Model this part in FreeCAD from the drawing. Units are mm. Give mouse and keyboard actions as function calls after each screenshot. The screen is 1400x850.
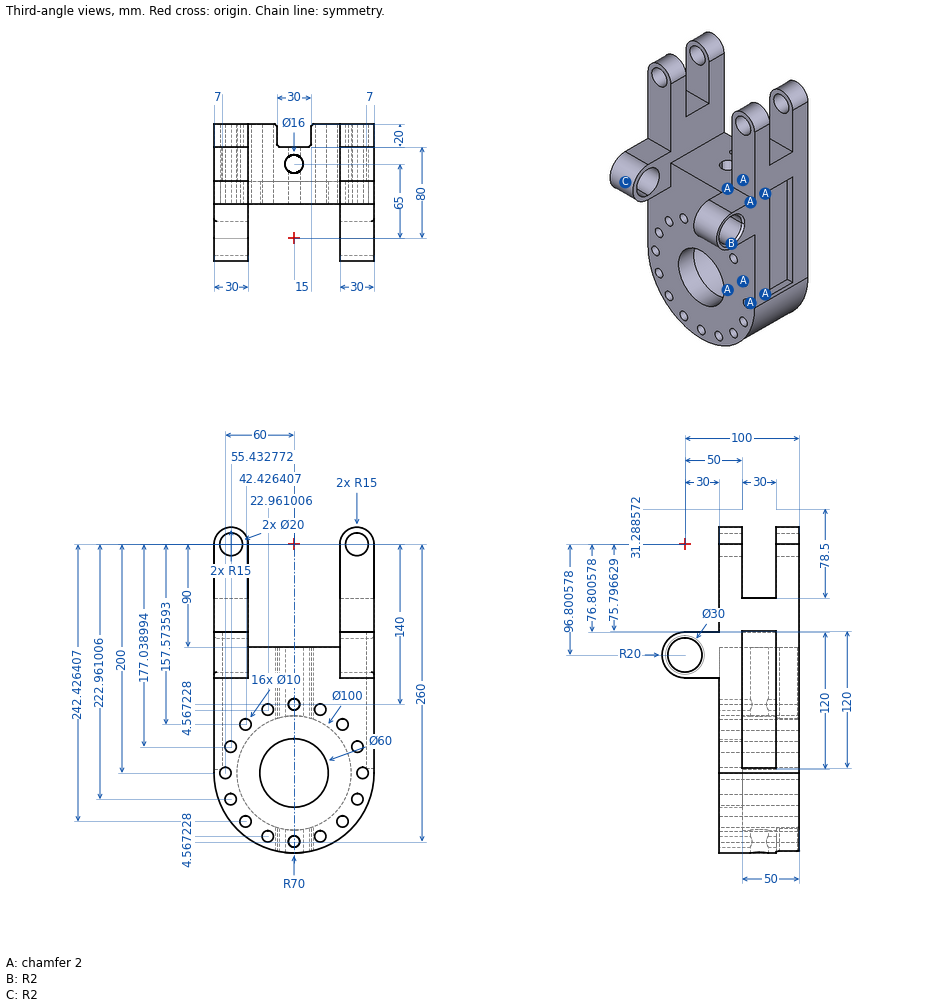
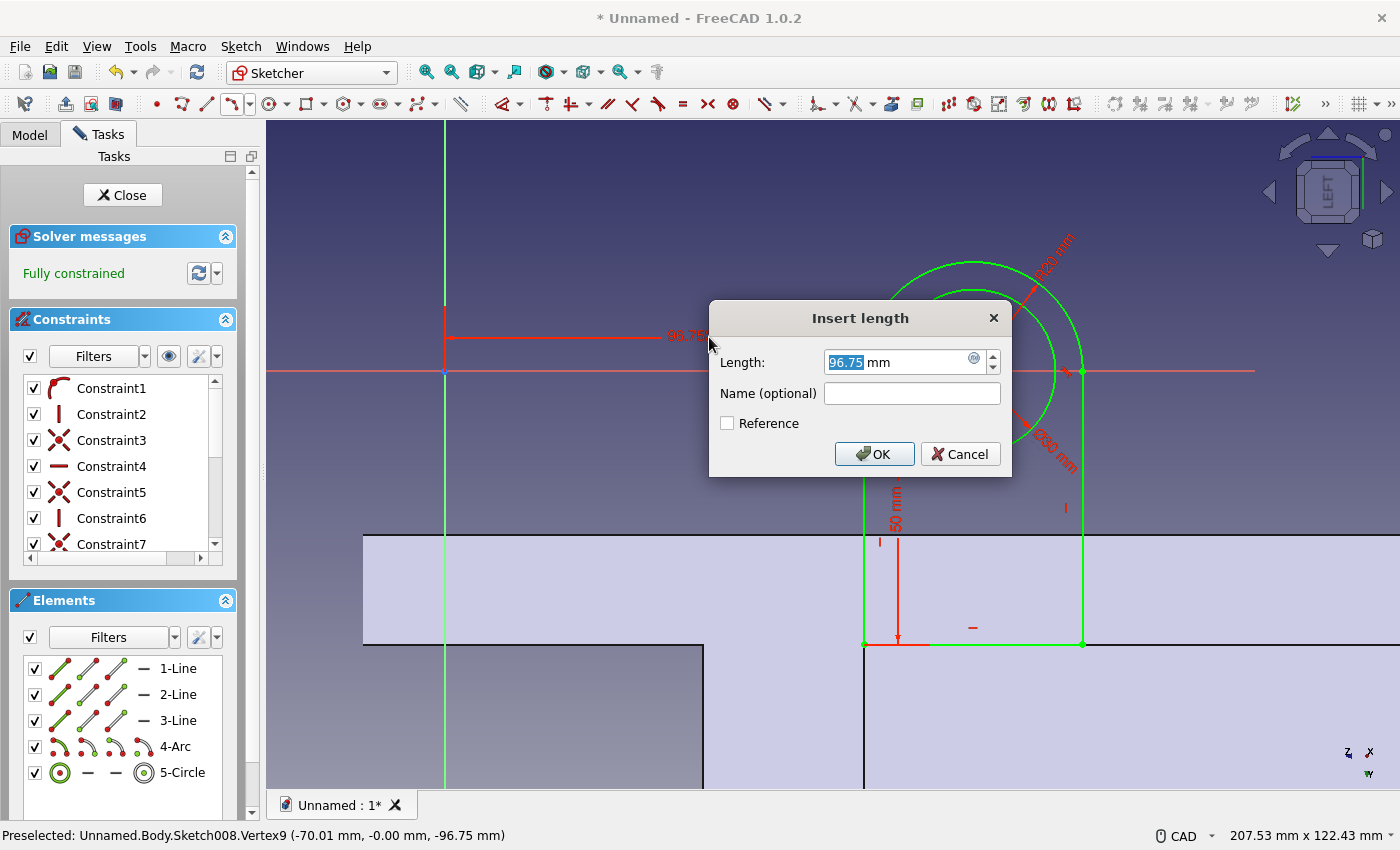
text(96.800578)
key(Return)
key(Escape)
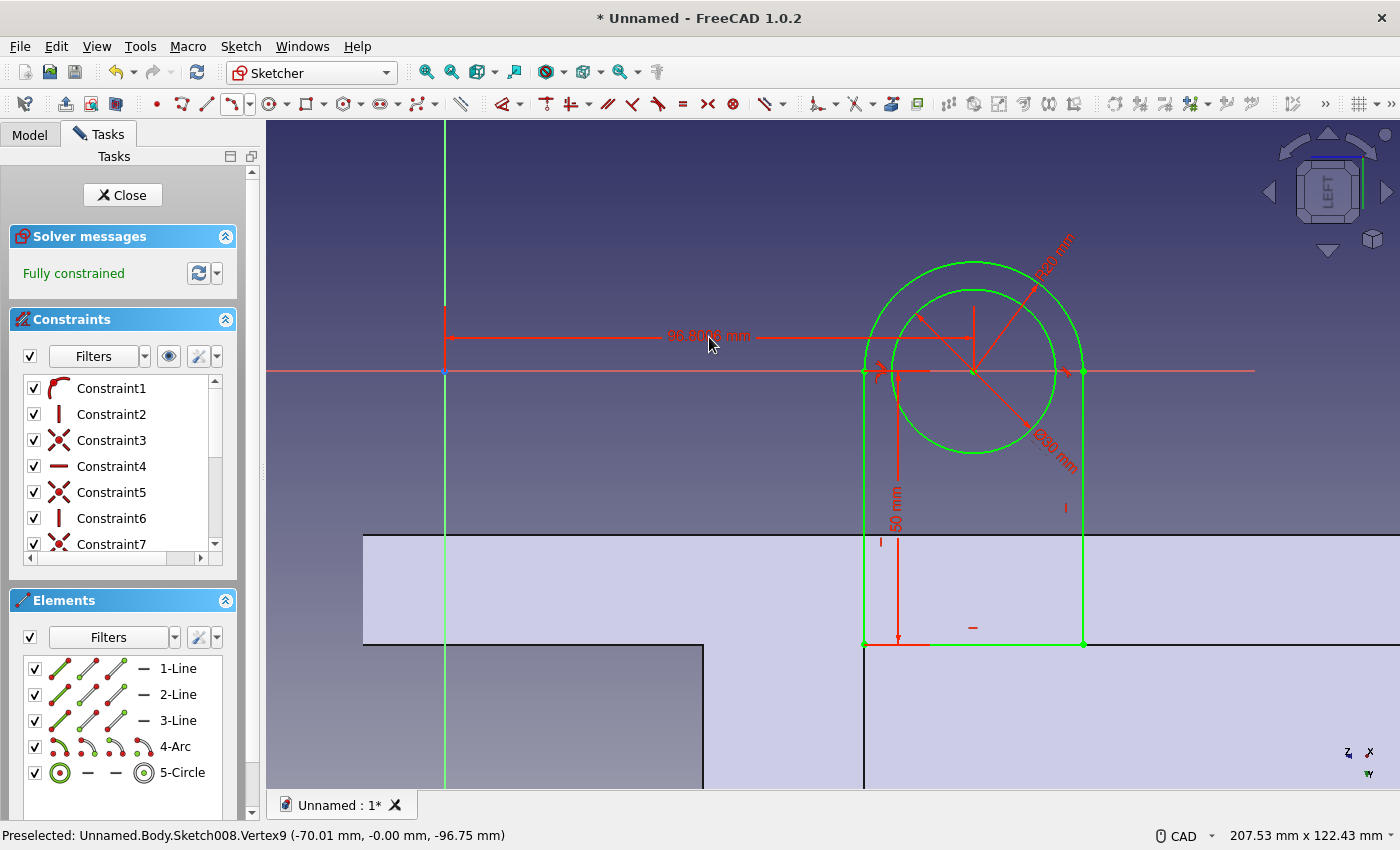
click(123, 195)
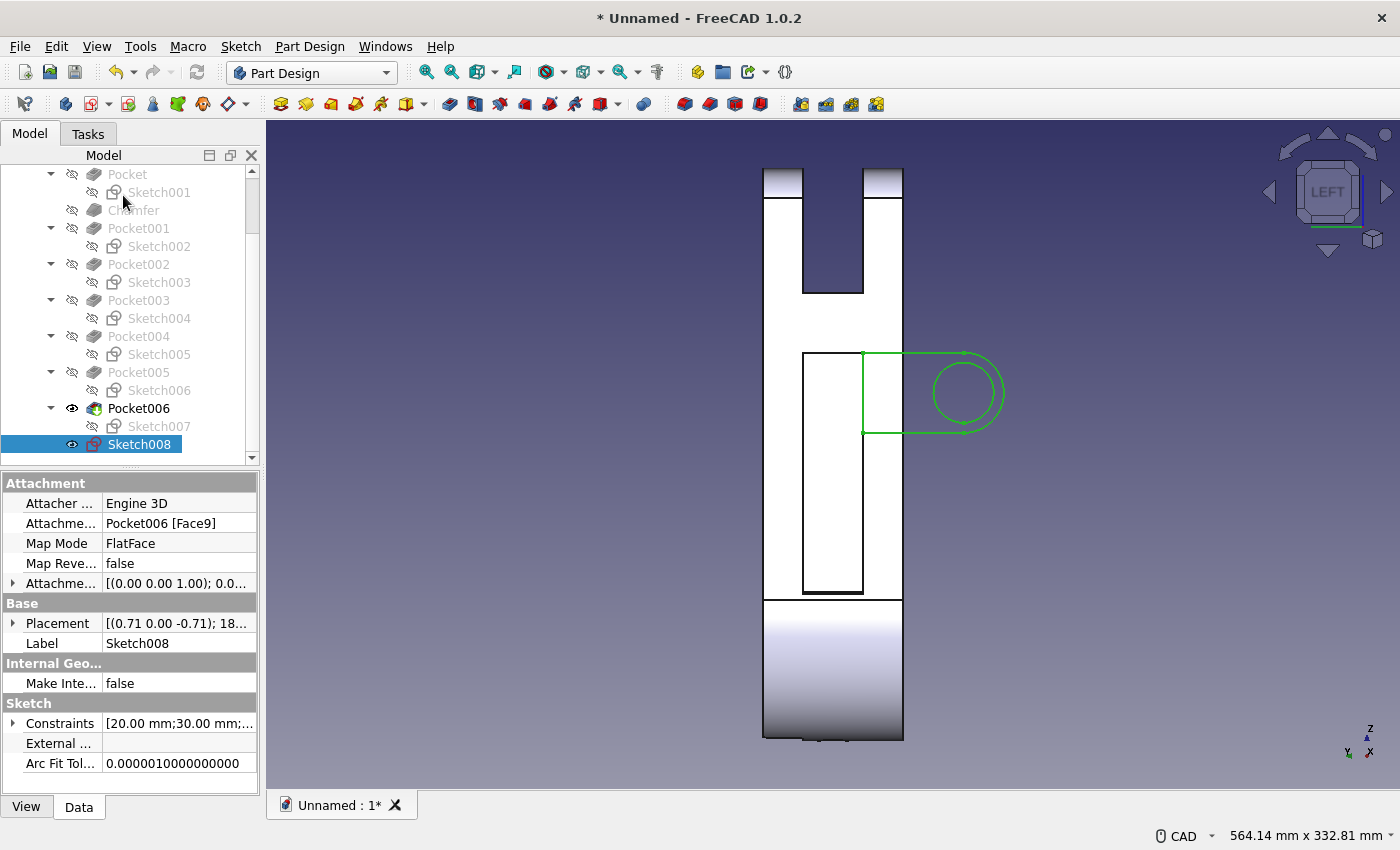
click(281, 104)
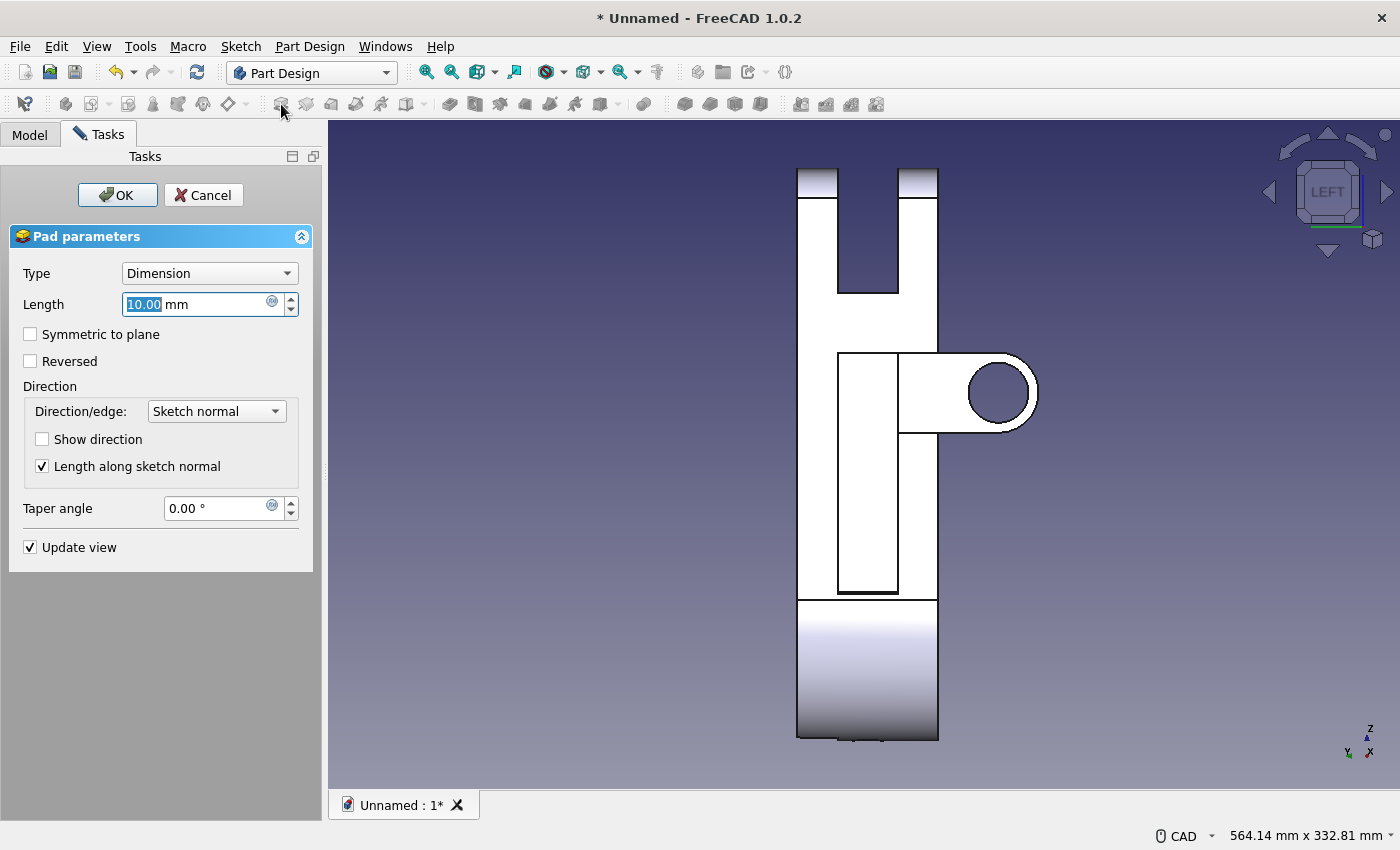
text(30)
key(Tab)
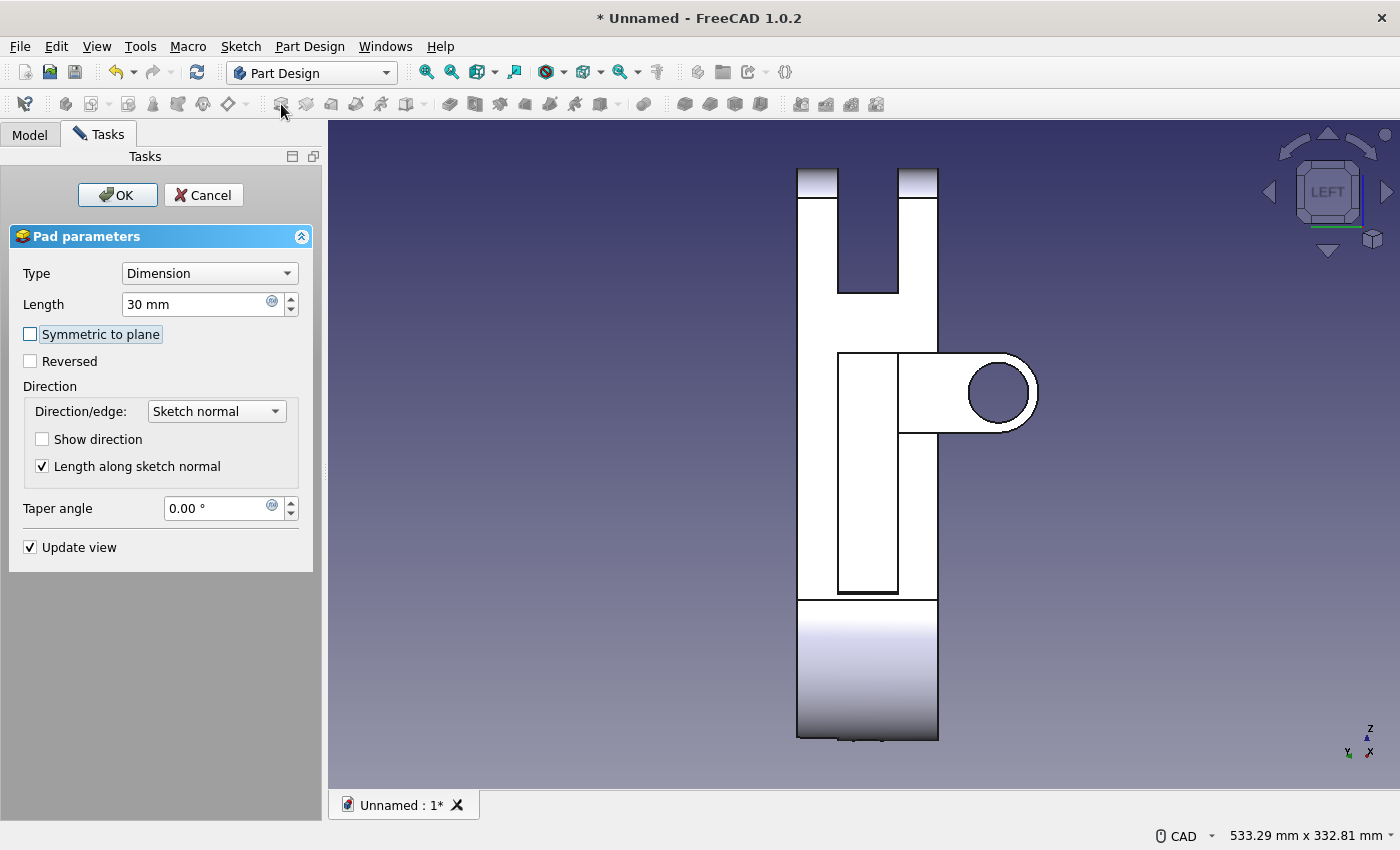
click(31, 361)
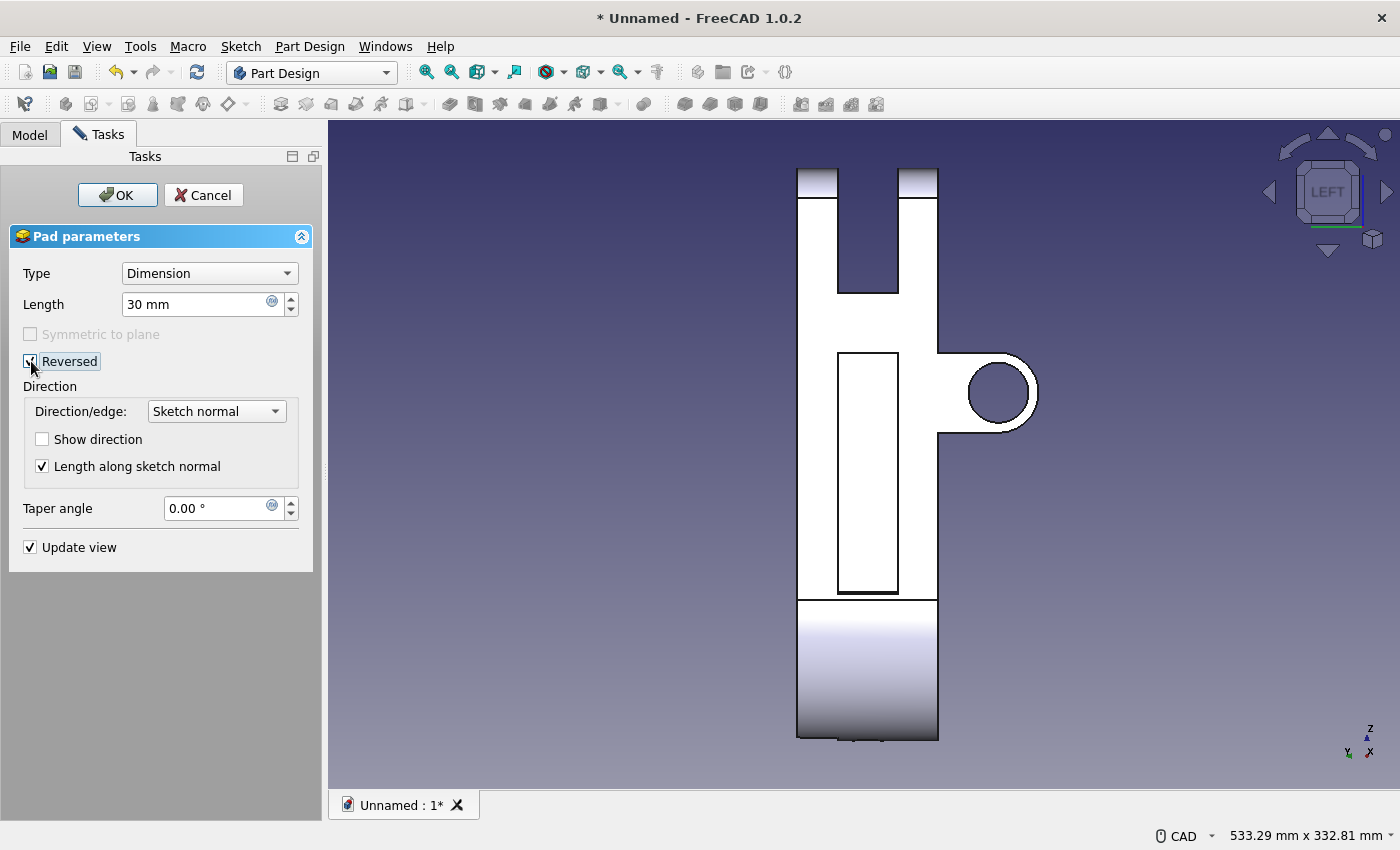
click(118, 195)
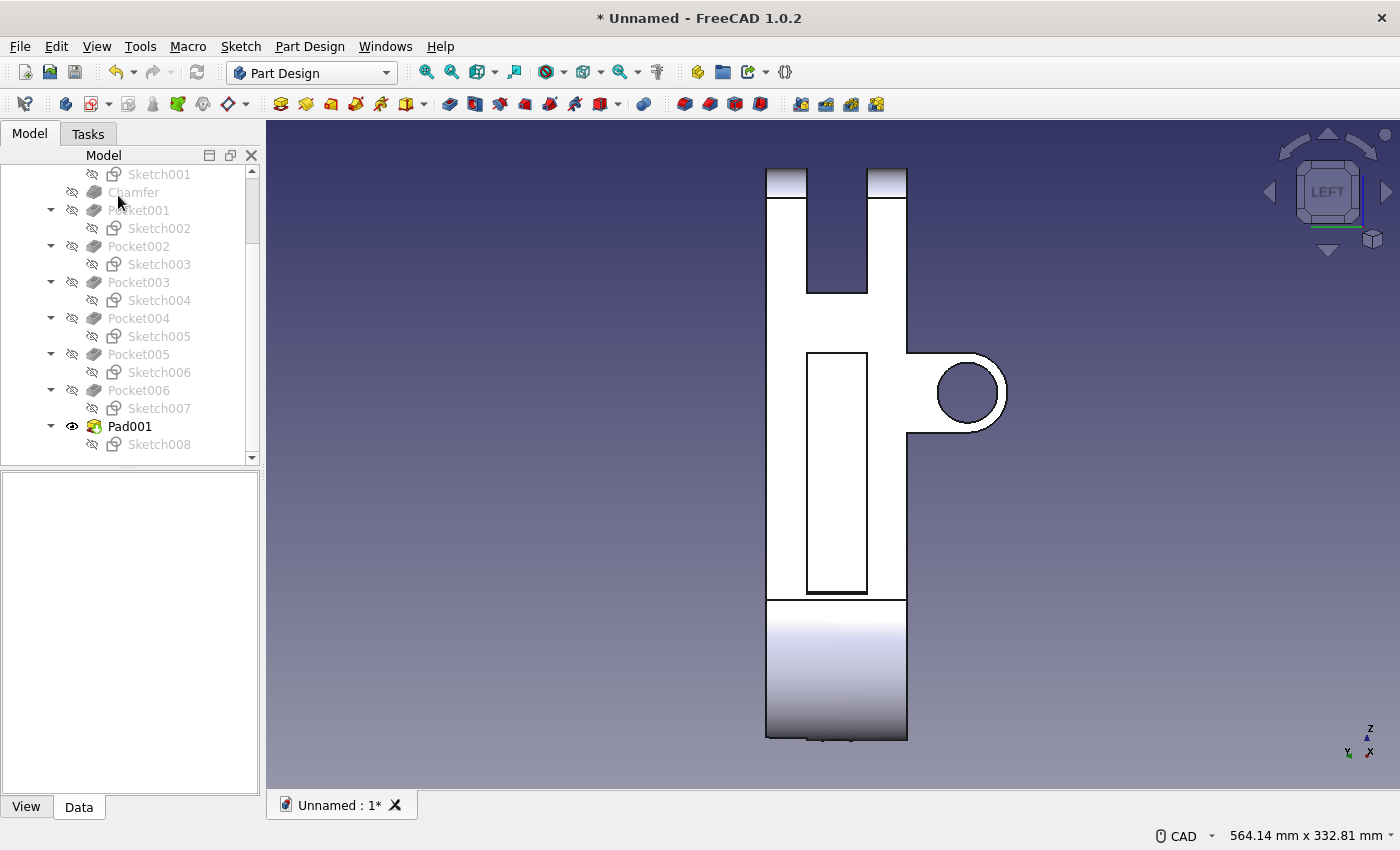
scroll(161, 314, down, 3)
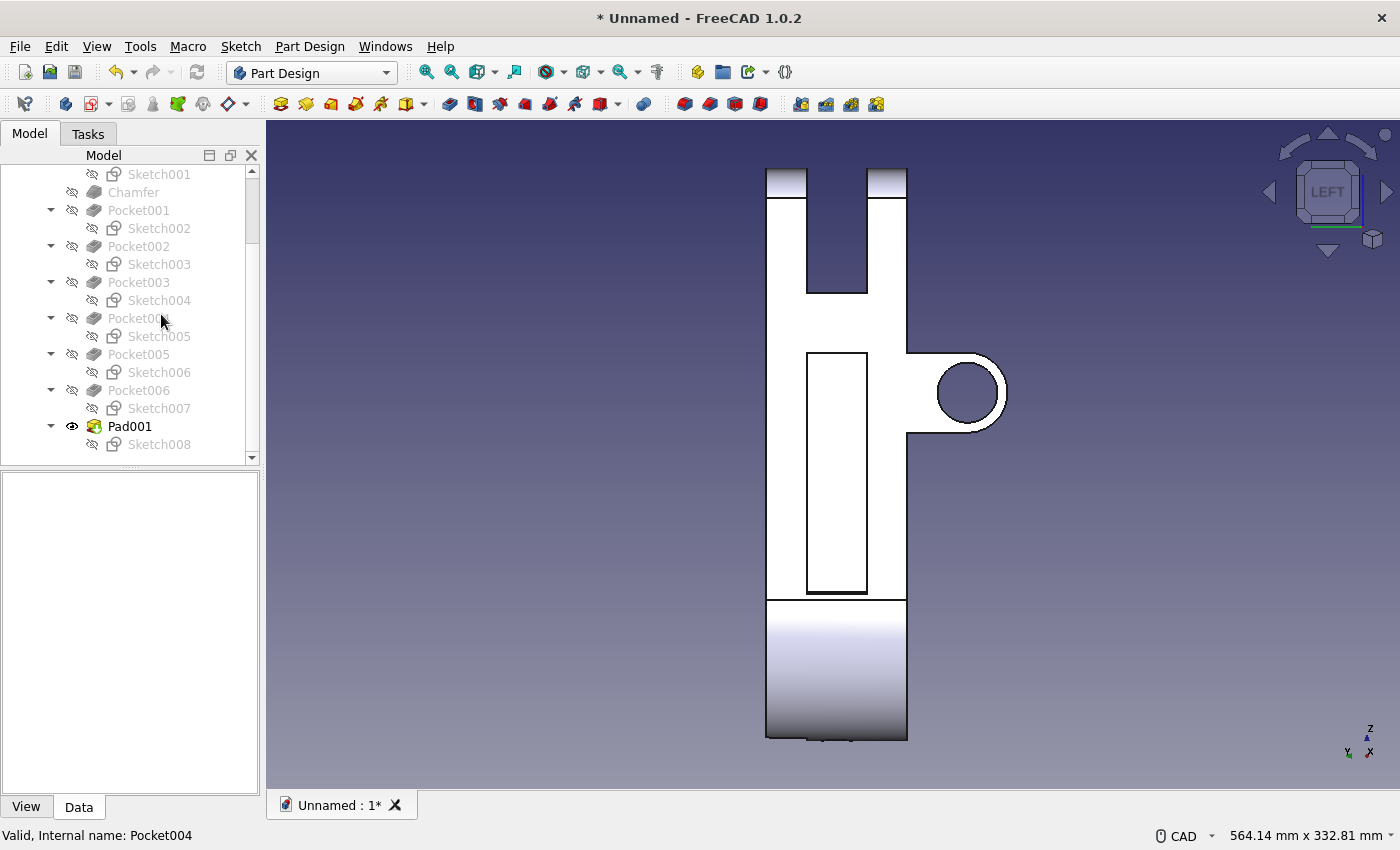
scroll(161, 314, up, 15)